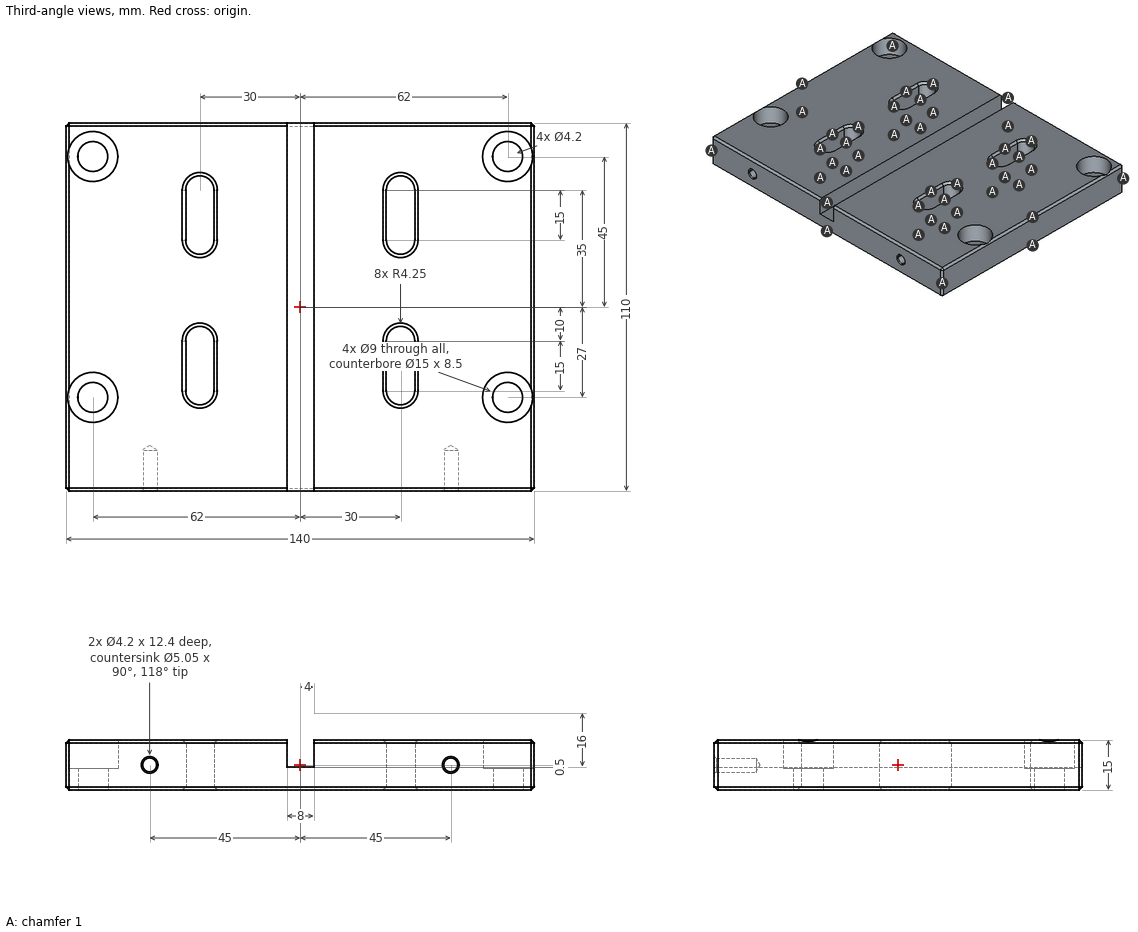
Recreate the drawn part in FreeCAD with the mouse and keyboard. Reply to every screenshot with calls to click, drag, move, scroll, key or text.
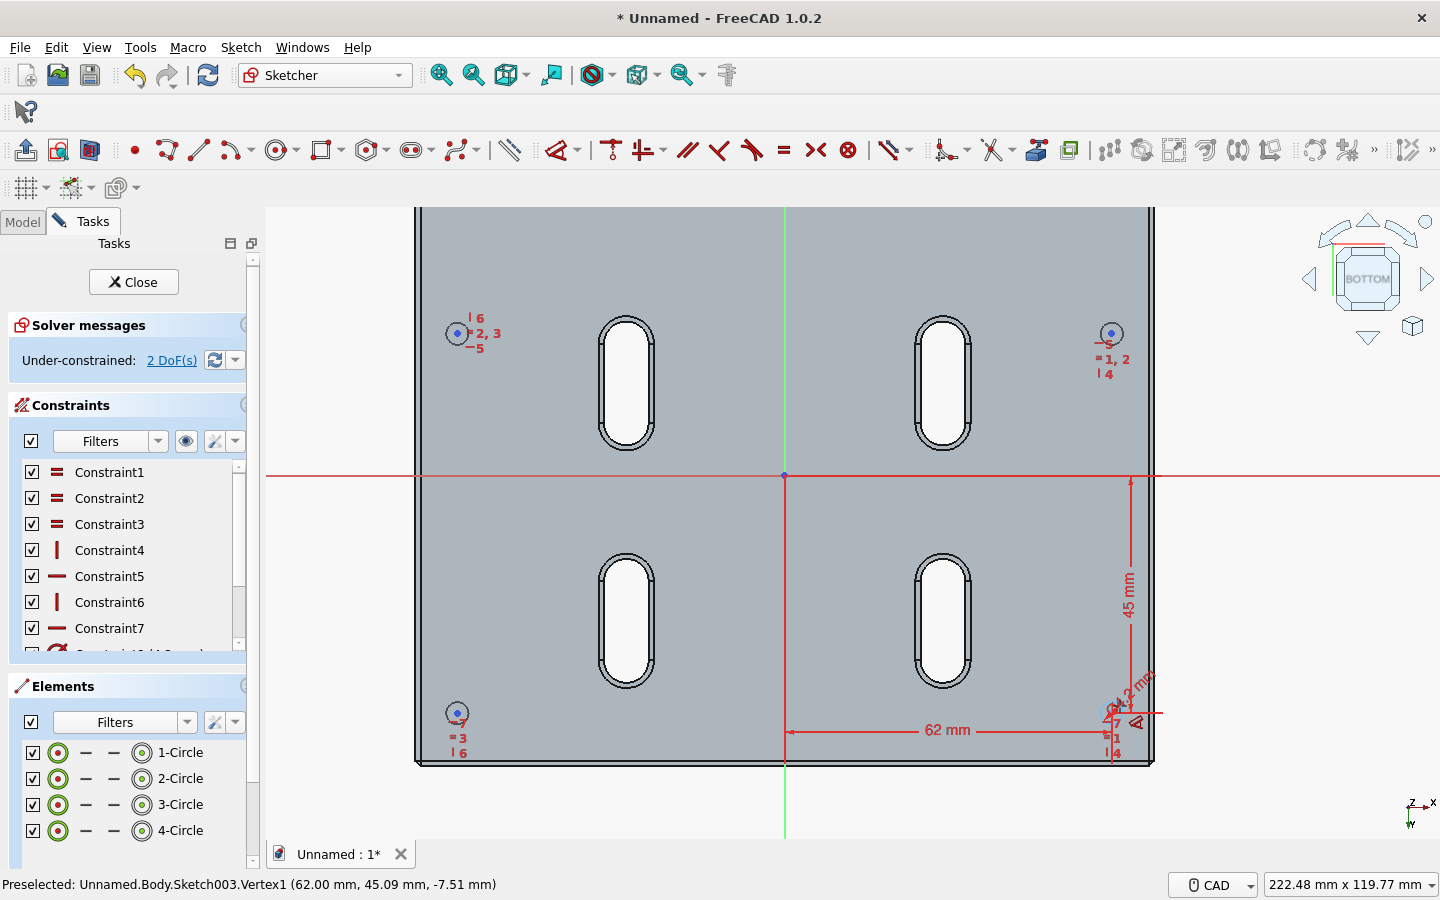
click(1112, 334)
click(1146, 405)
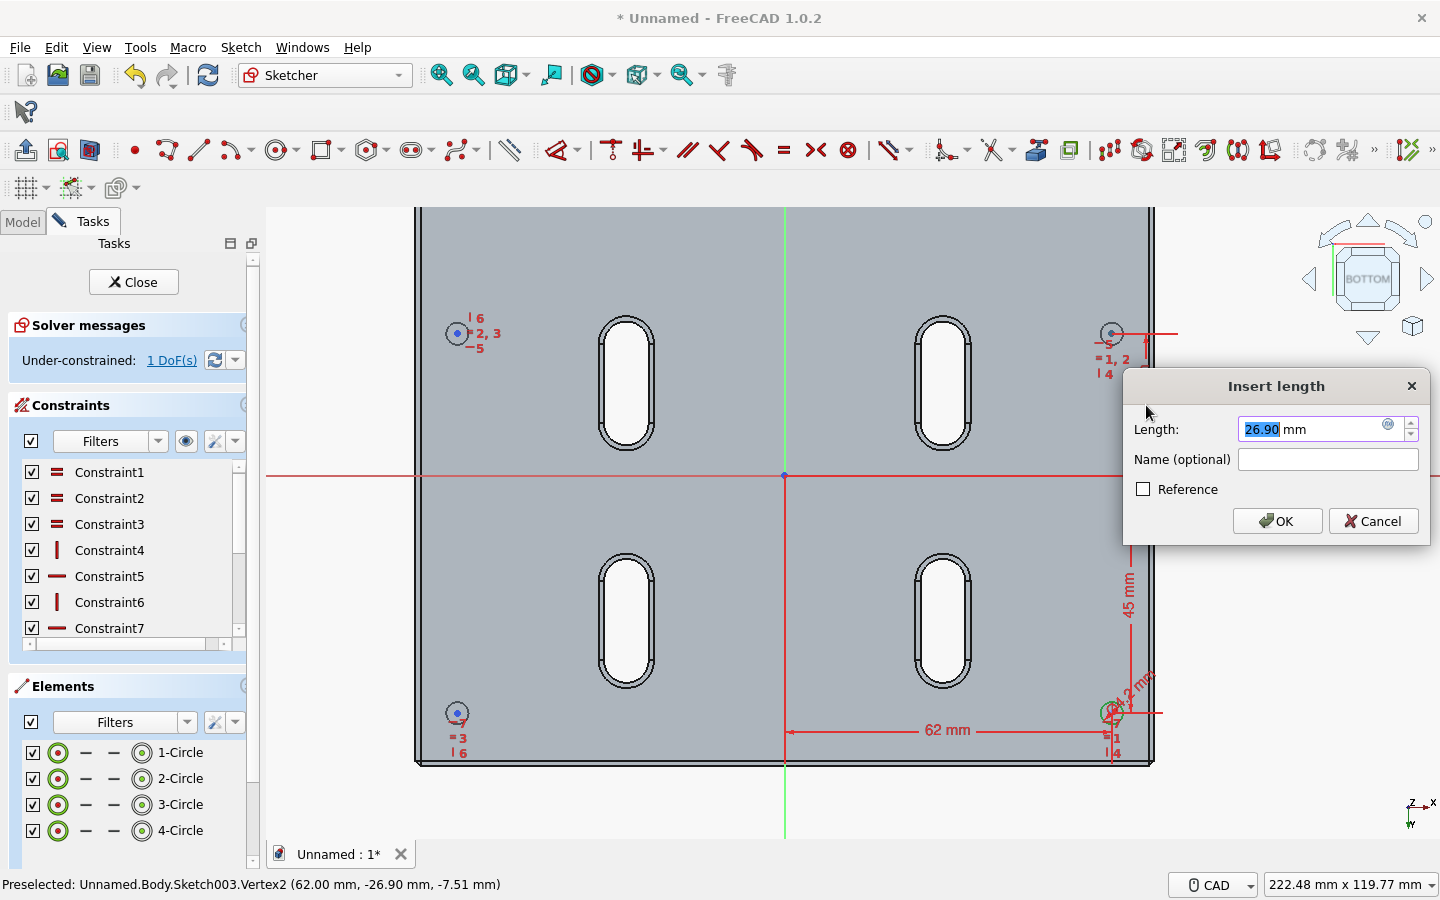
text(27)
key(Return)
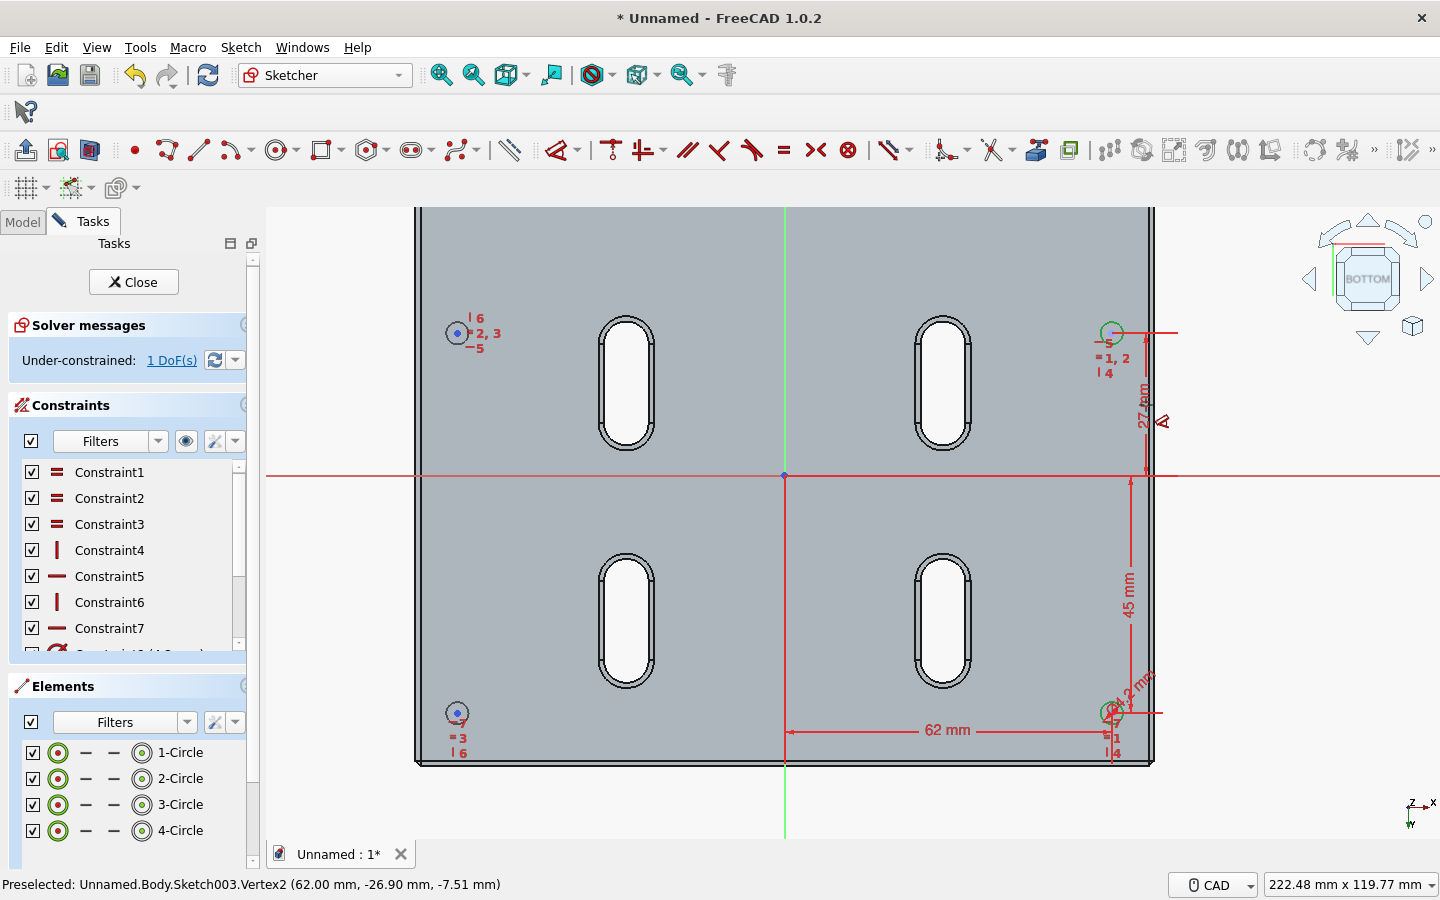
click(457, 333)
click(621, 299)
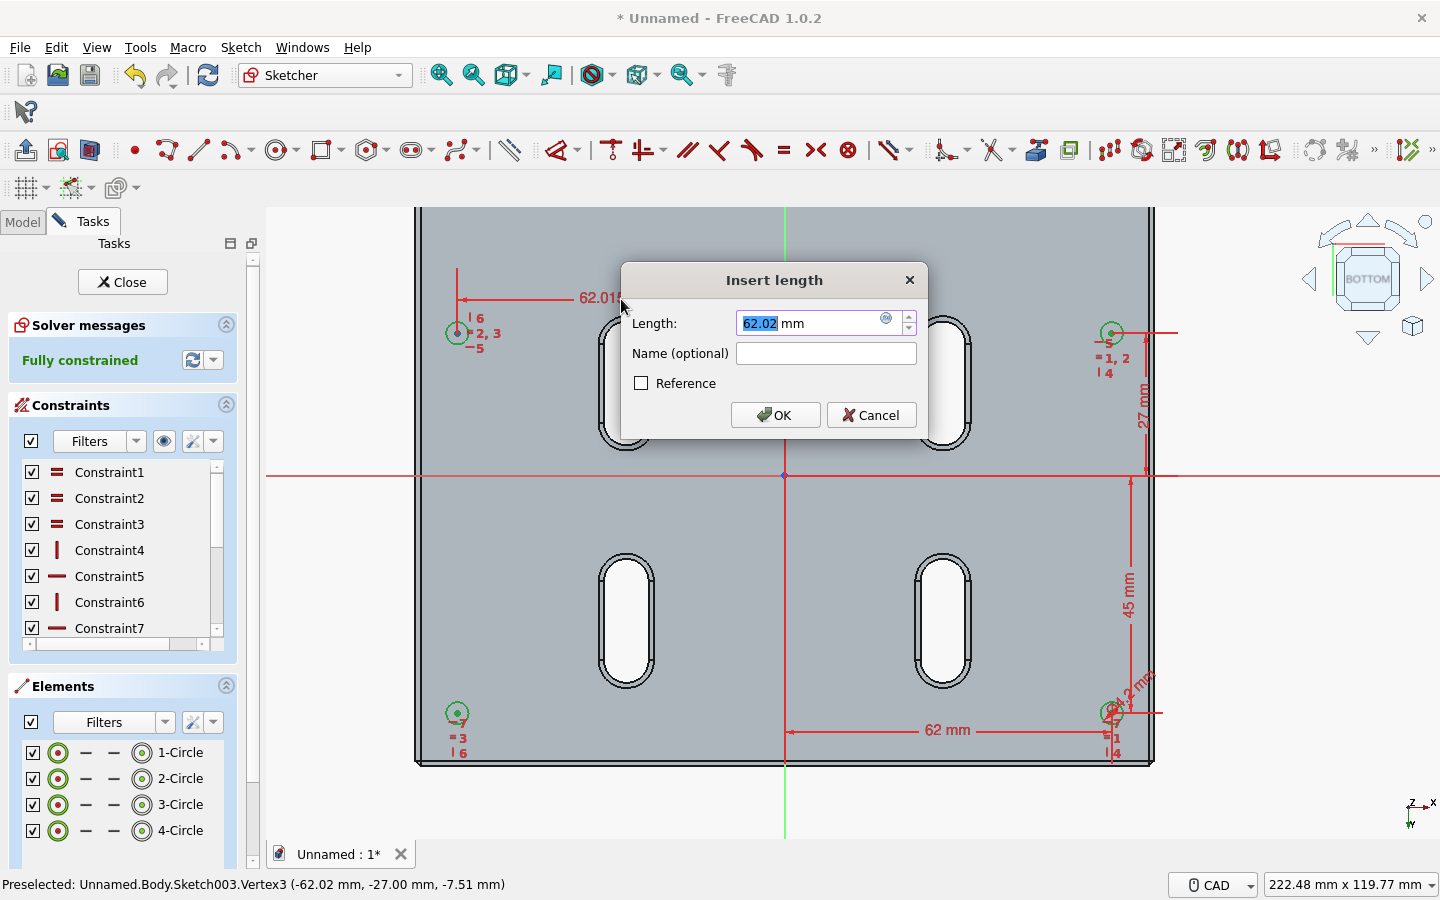
text(62)
key(Return)
key(Escape)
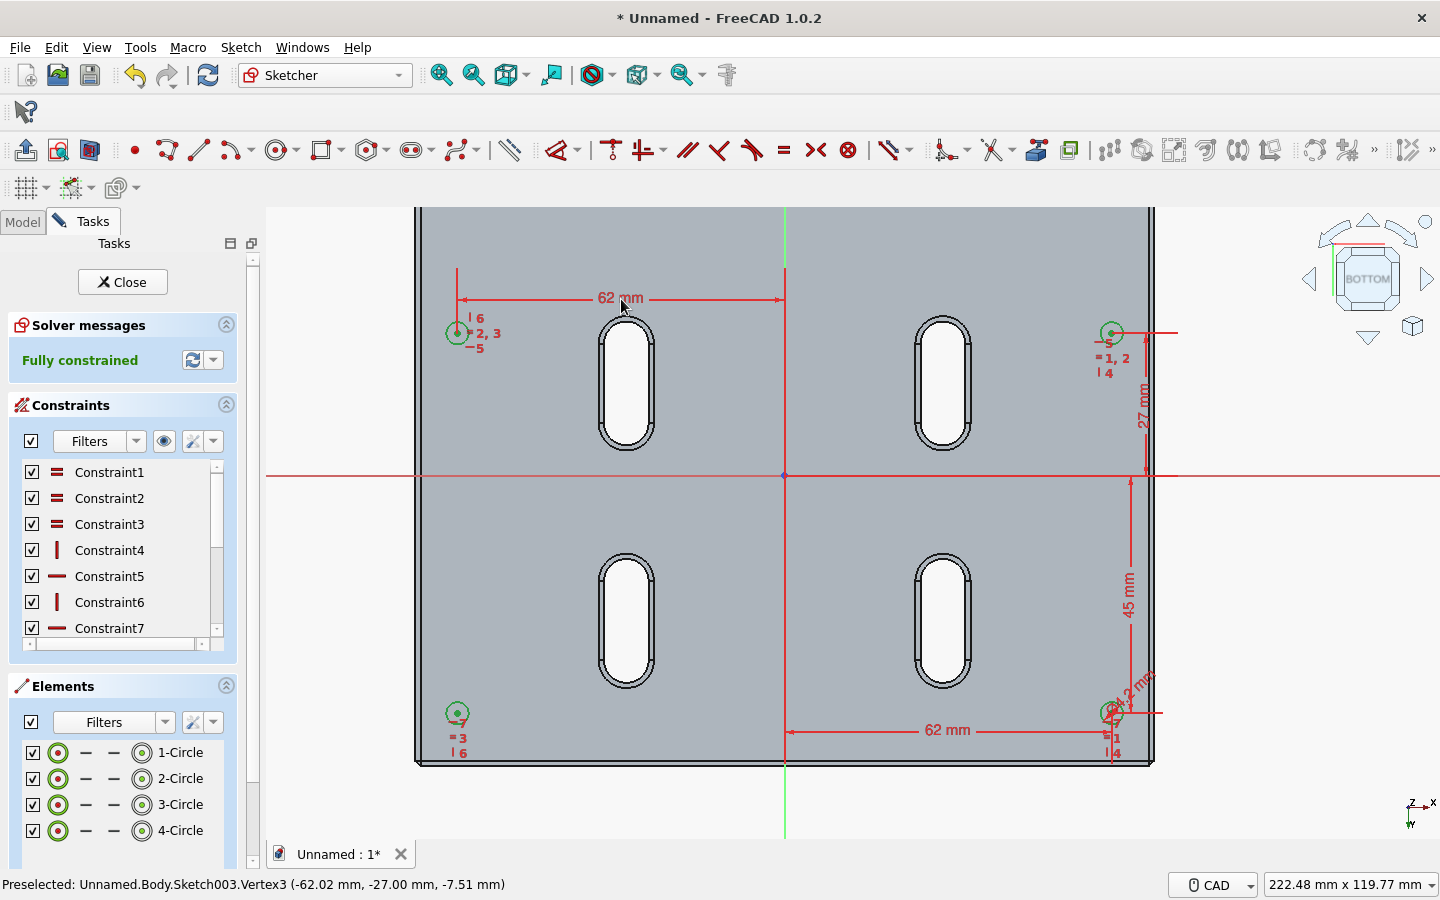
click(123, 282)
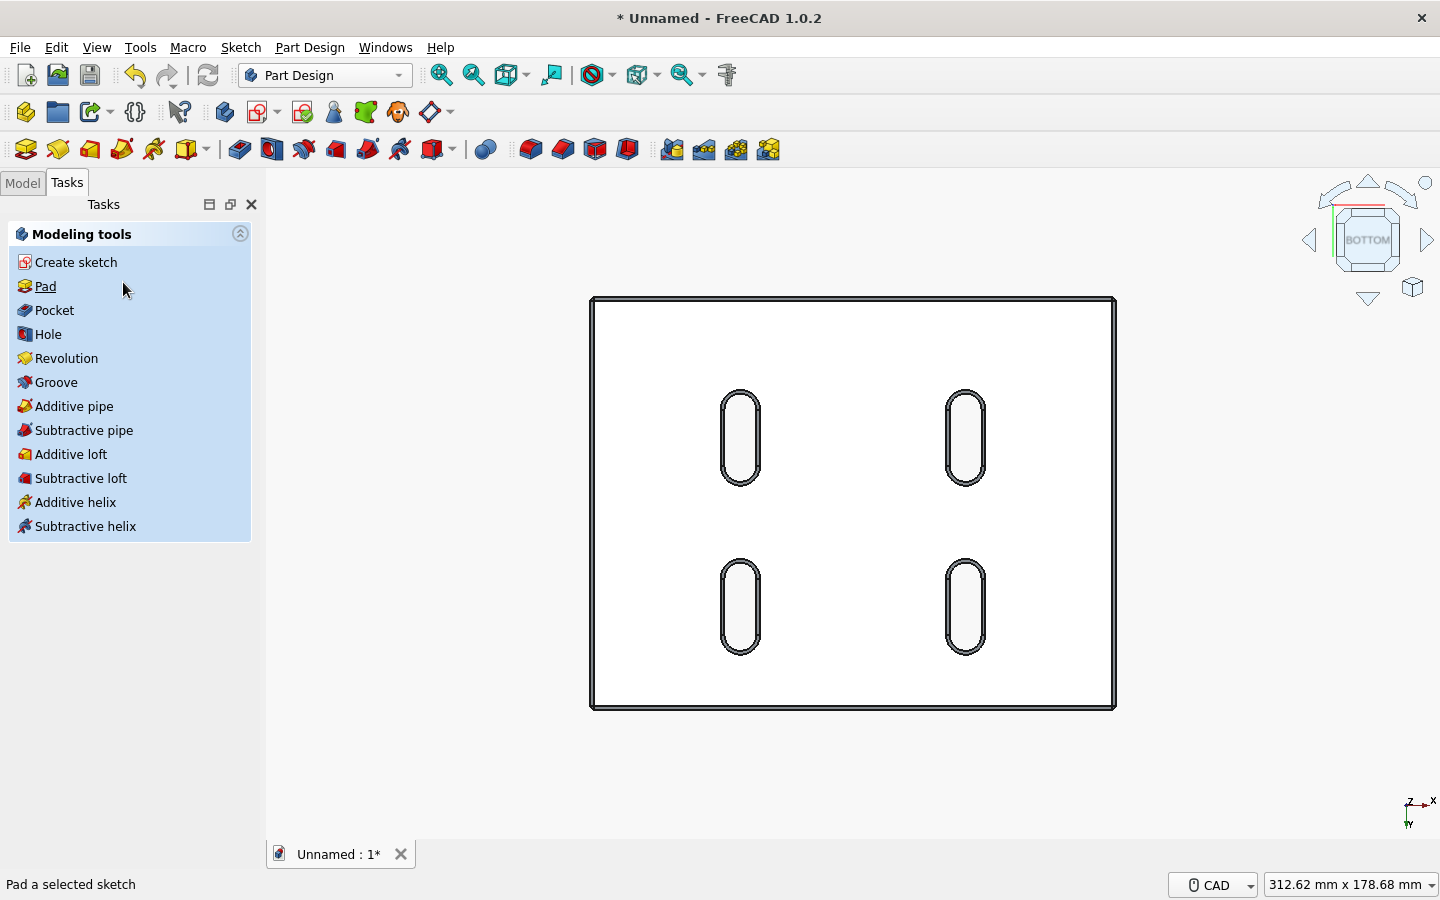
click(240, 150)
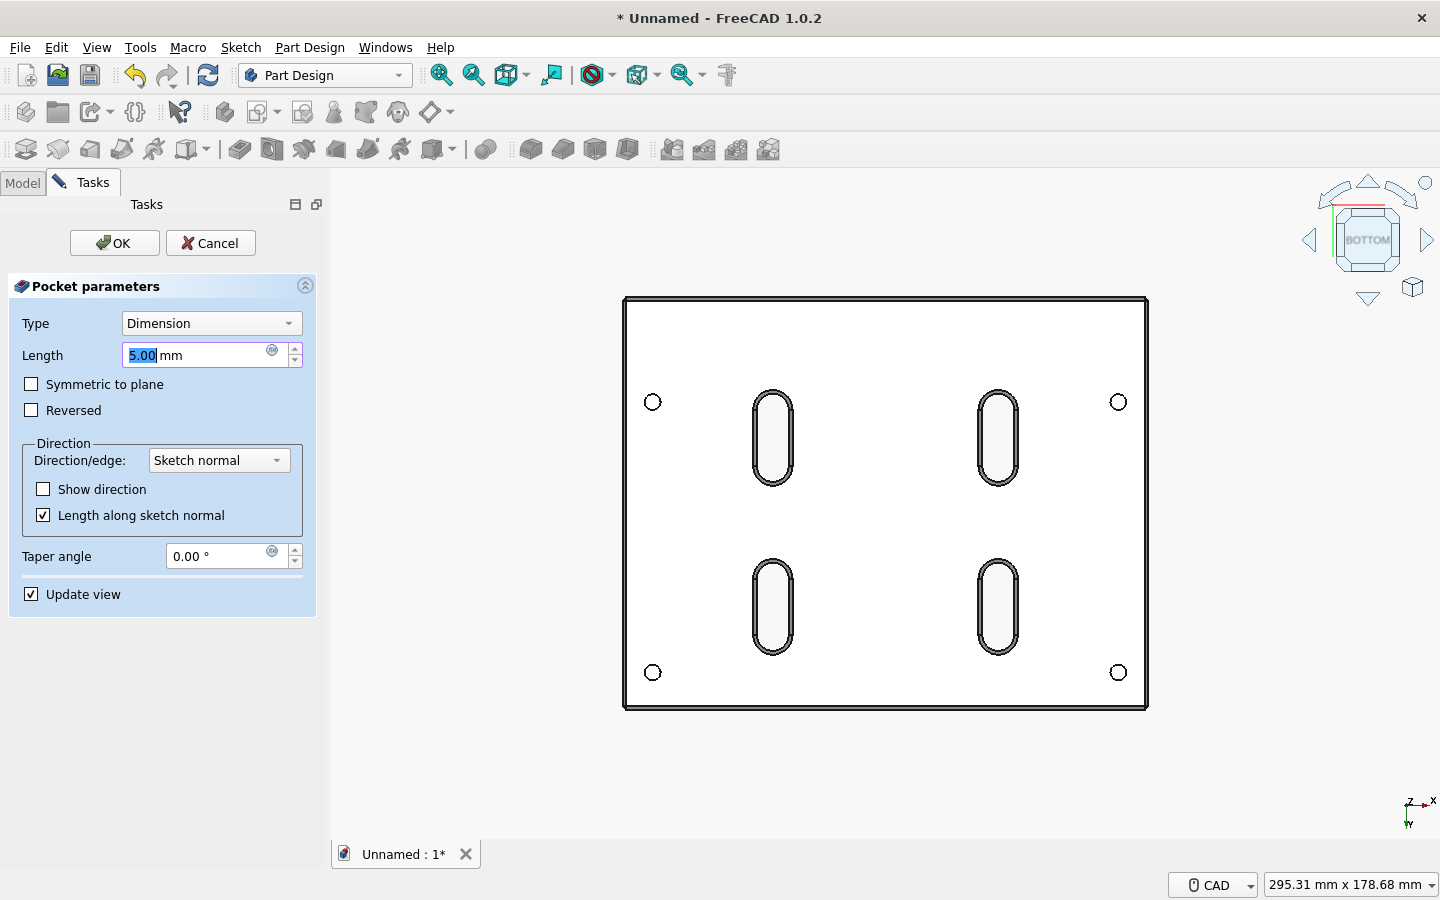
click(212, 324)